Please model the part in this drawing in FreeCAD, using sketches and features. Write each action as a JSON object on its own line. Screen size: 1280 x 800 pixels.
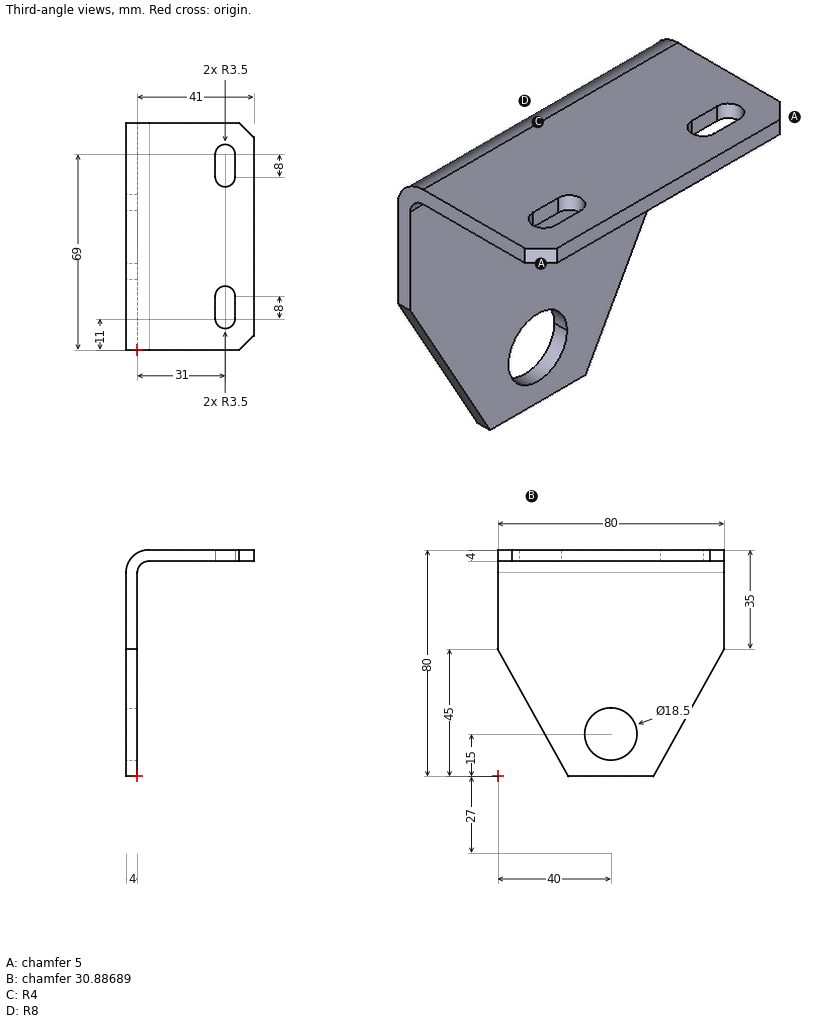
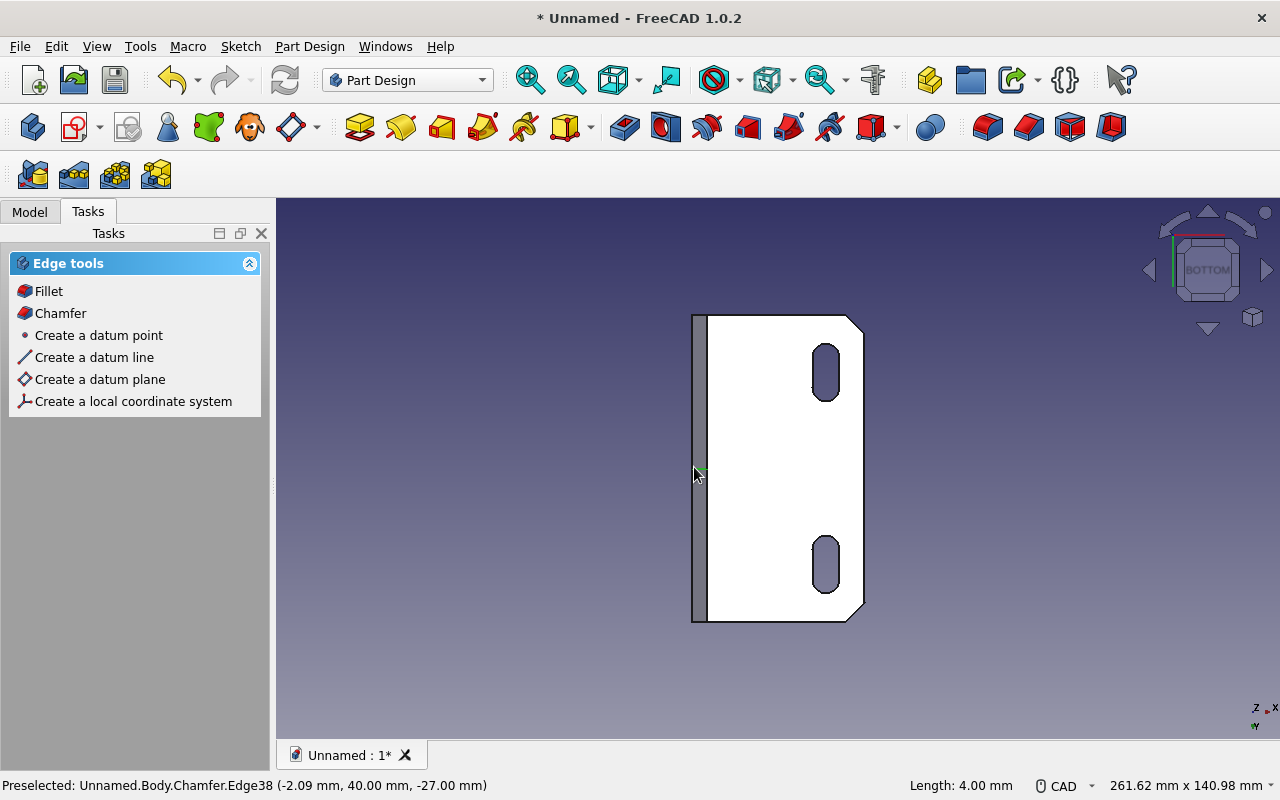
{"action": "left_click", "coordinate": [1029, 128]}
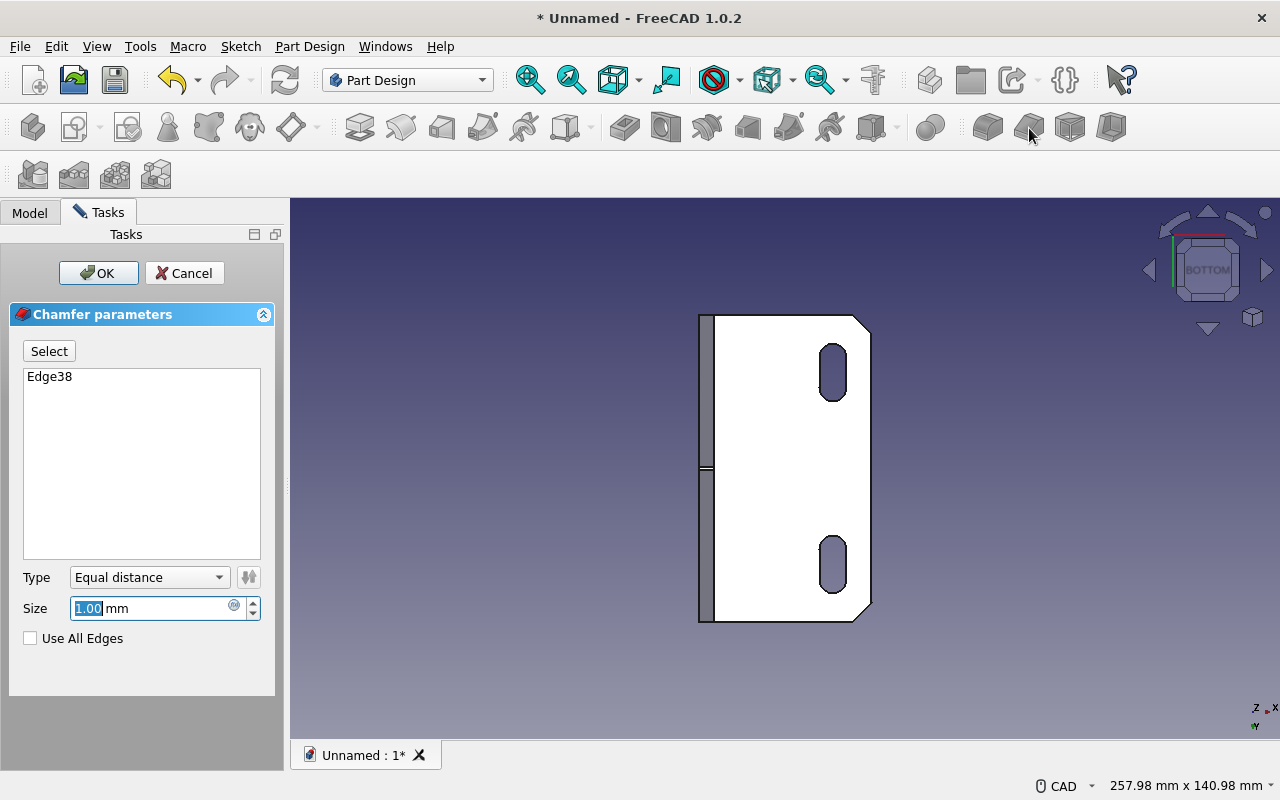
{"action": "type", "text": "30.88689"}
{"action": "key", "text": "Tab"}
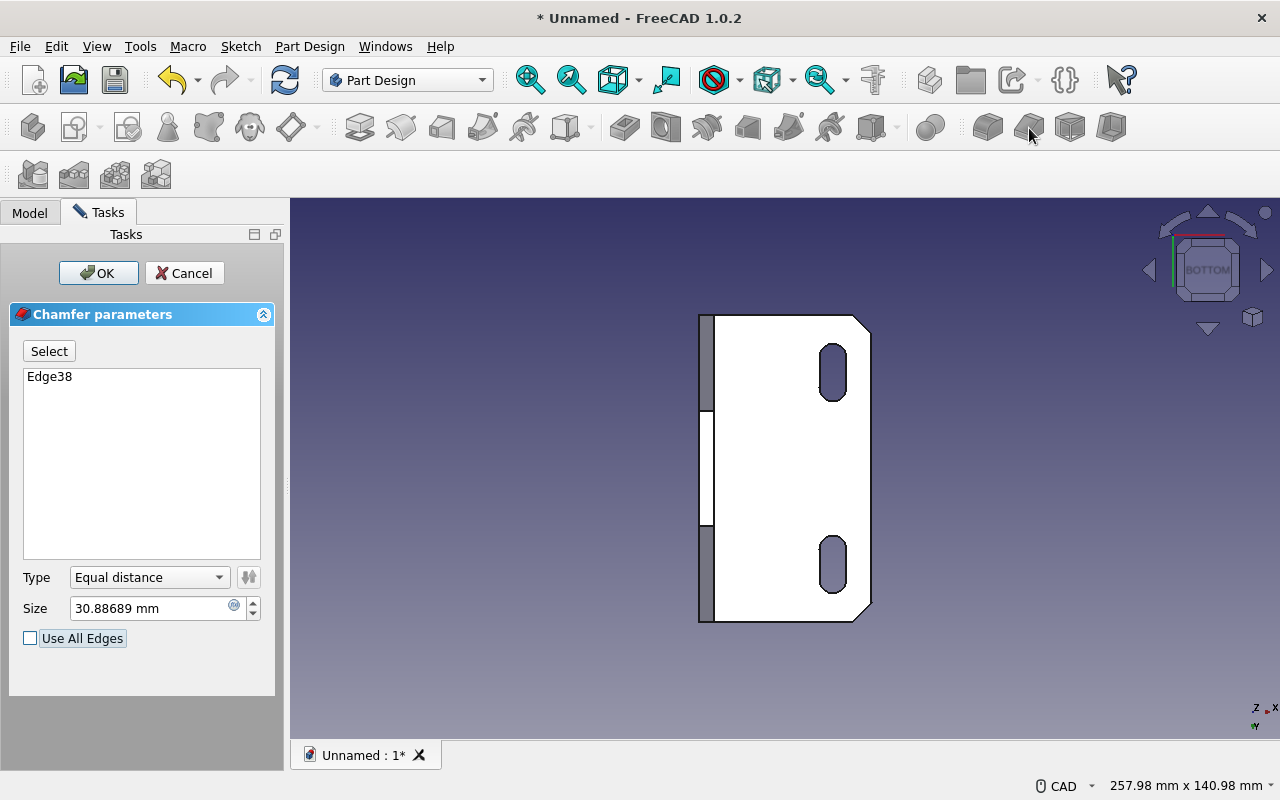
{"action": "left_click", "coordinate": [99, 273]}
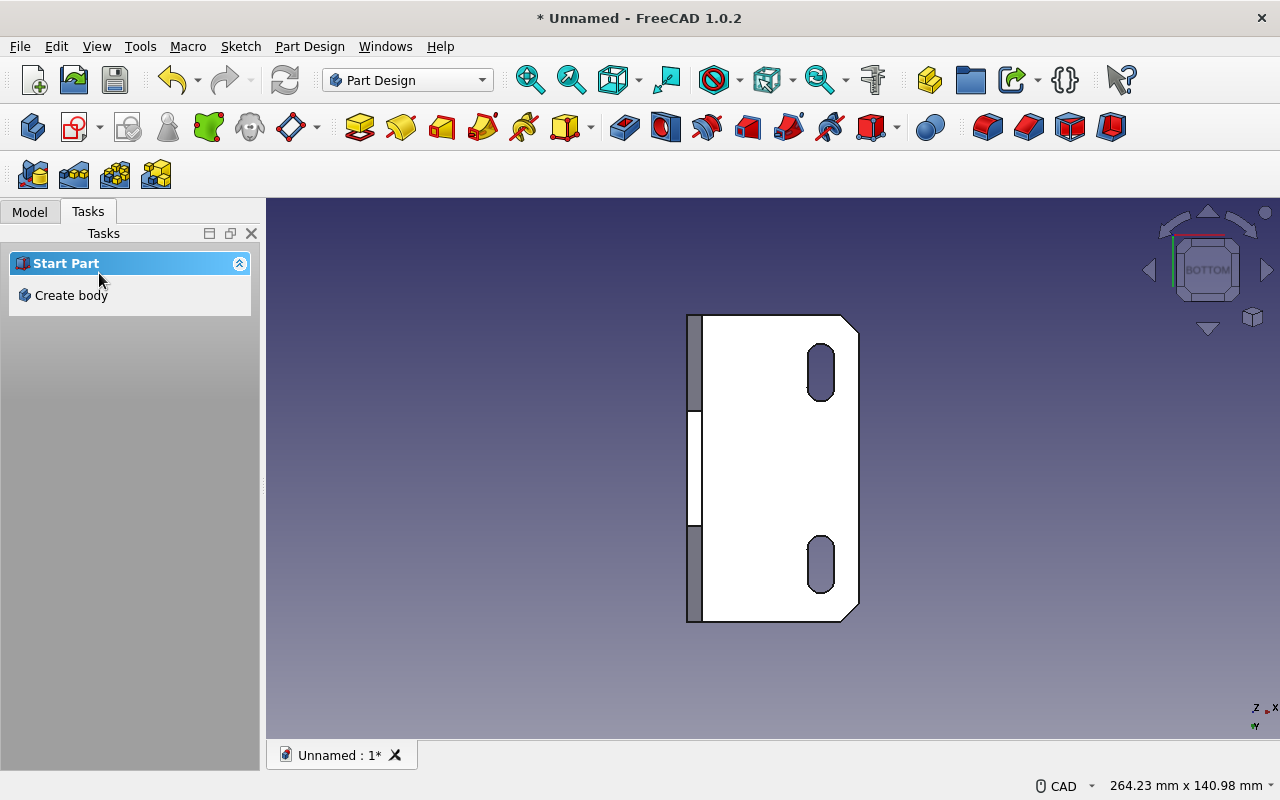
{"action": "key", "text": "0"}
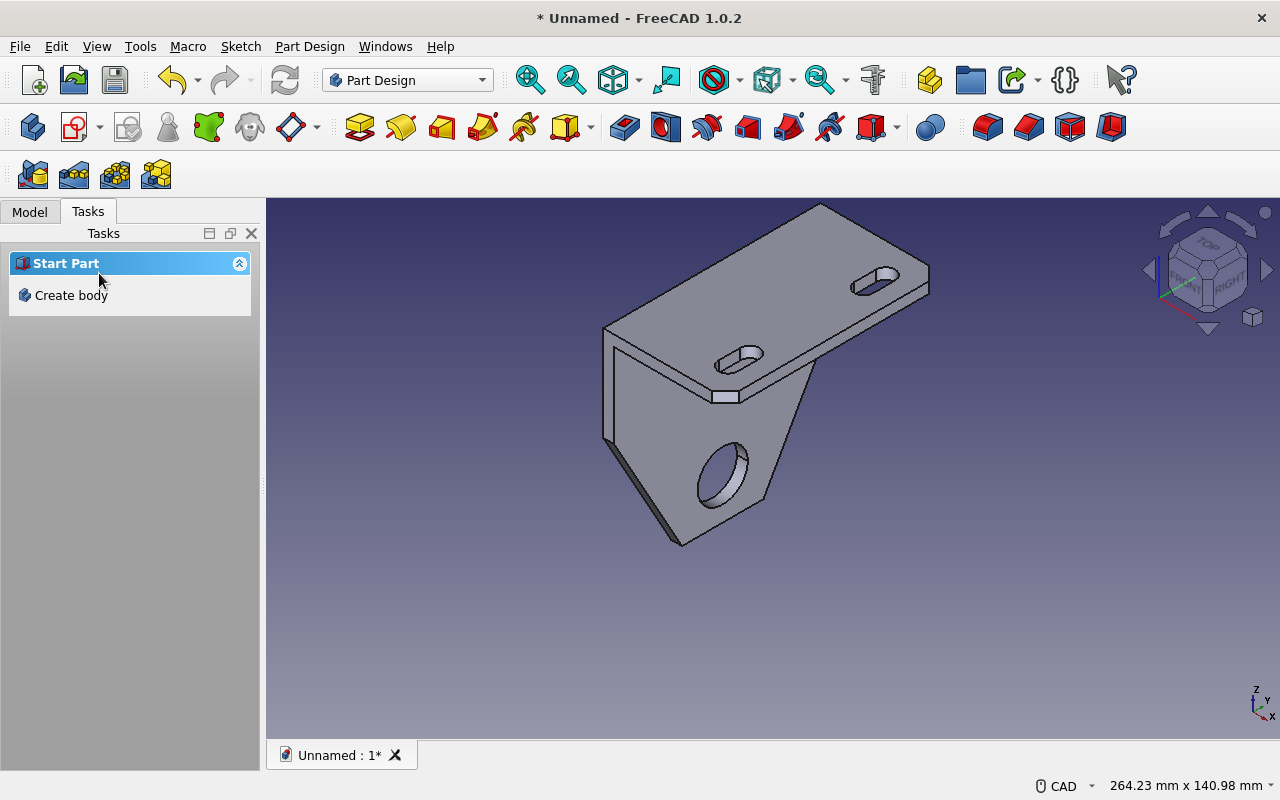
{"action": "key", "text": "2"}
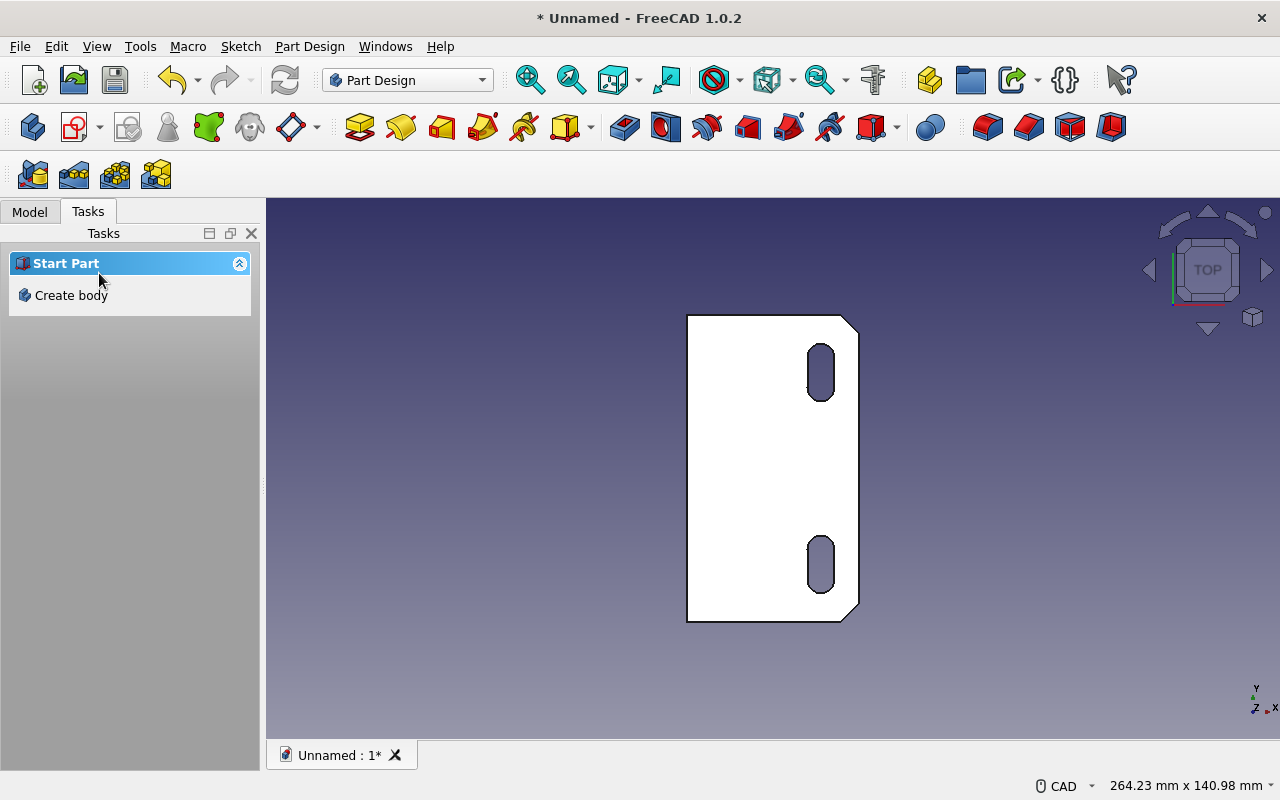
{"action": "key", "text": "1"}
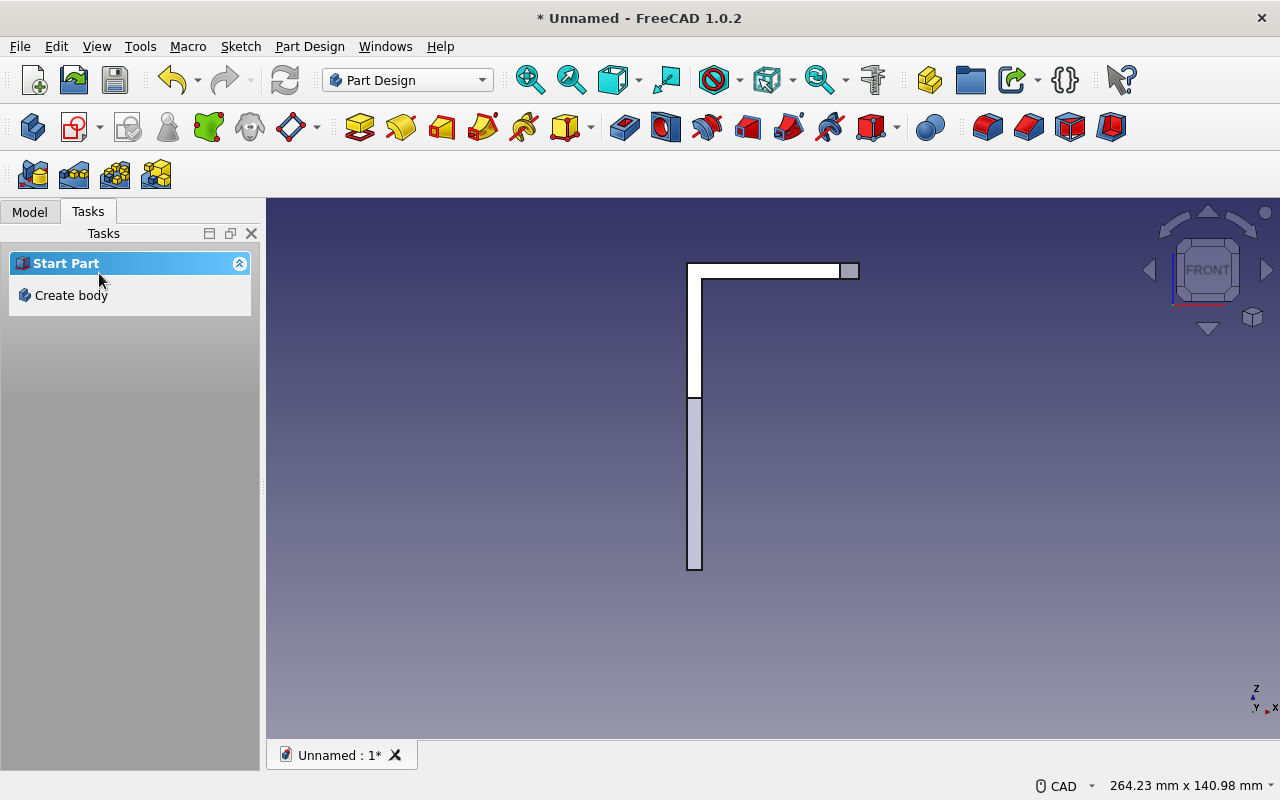
{"action": "key", "text": "3"}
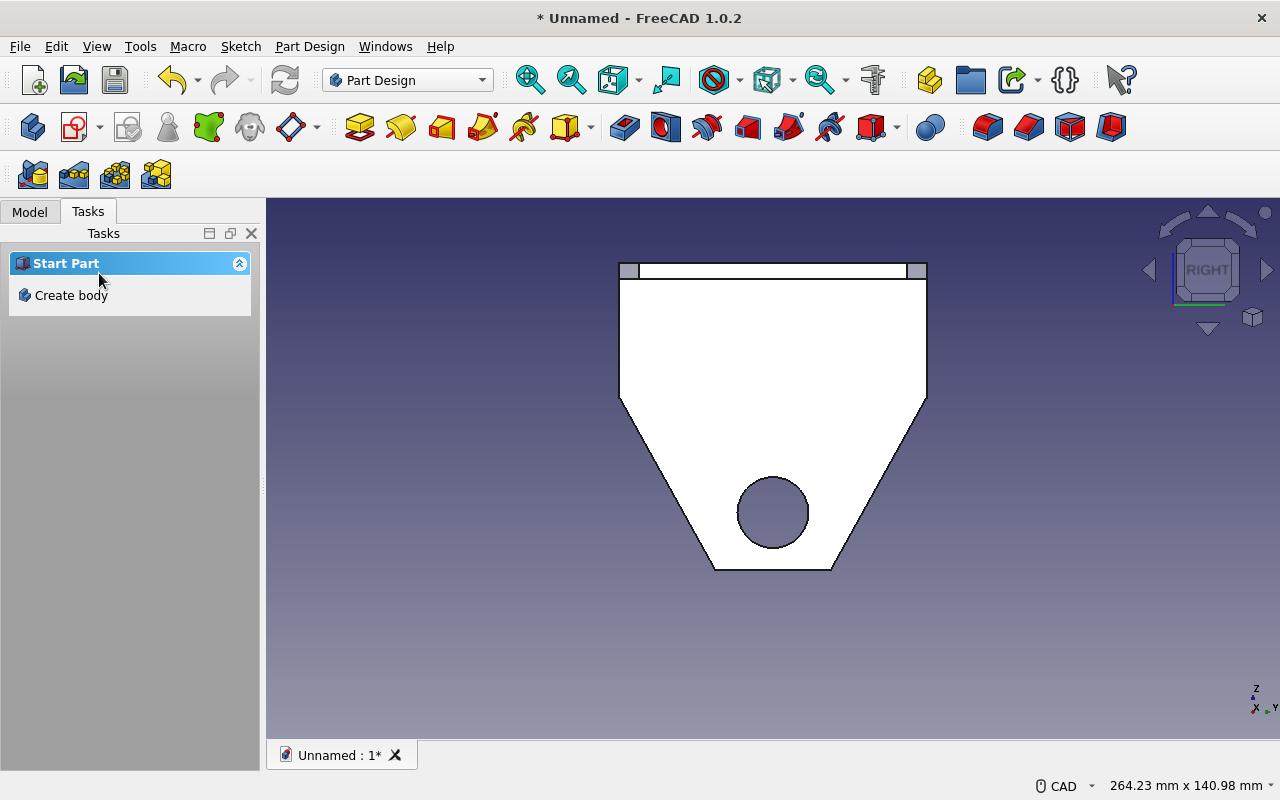
{"action": "key", "text": "5"}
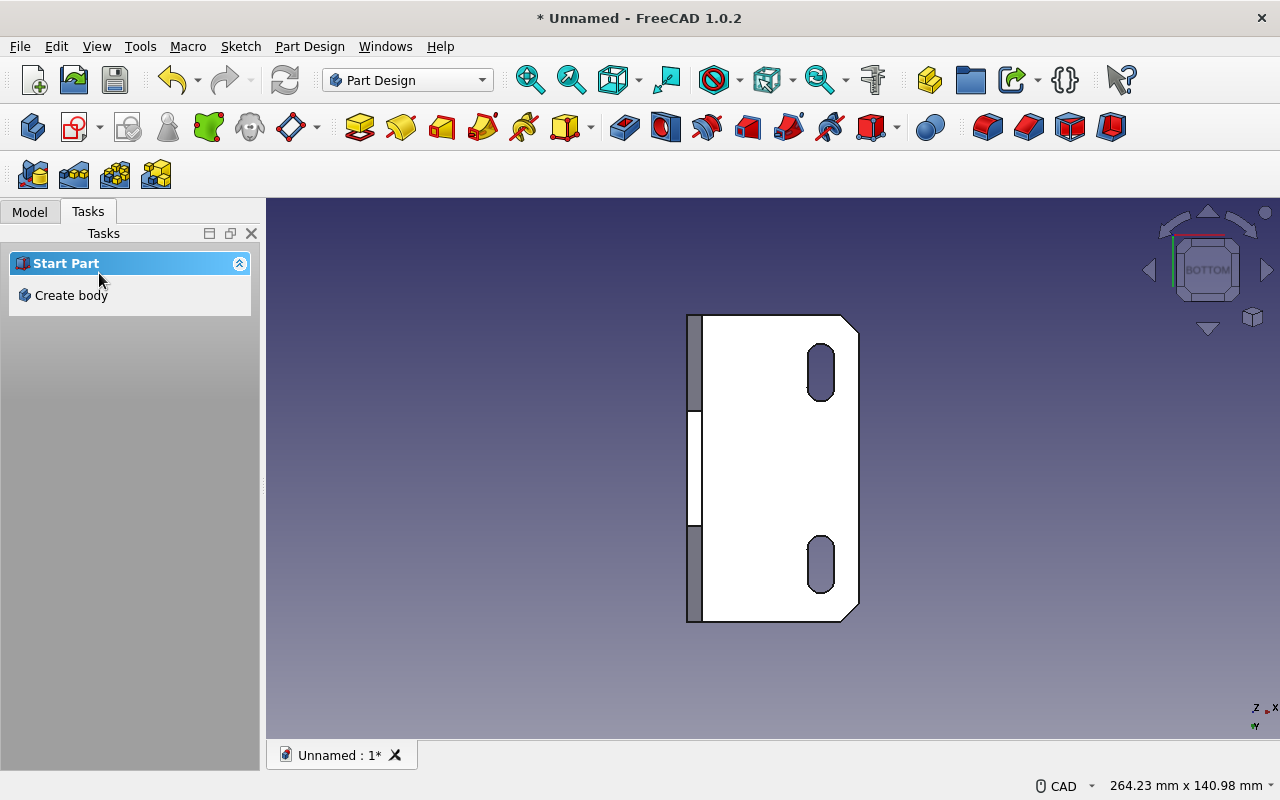
{"action": "key", "text": "4"}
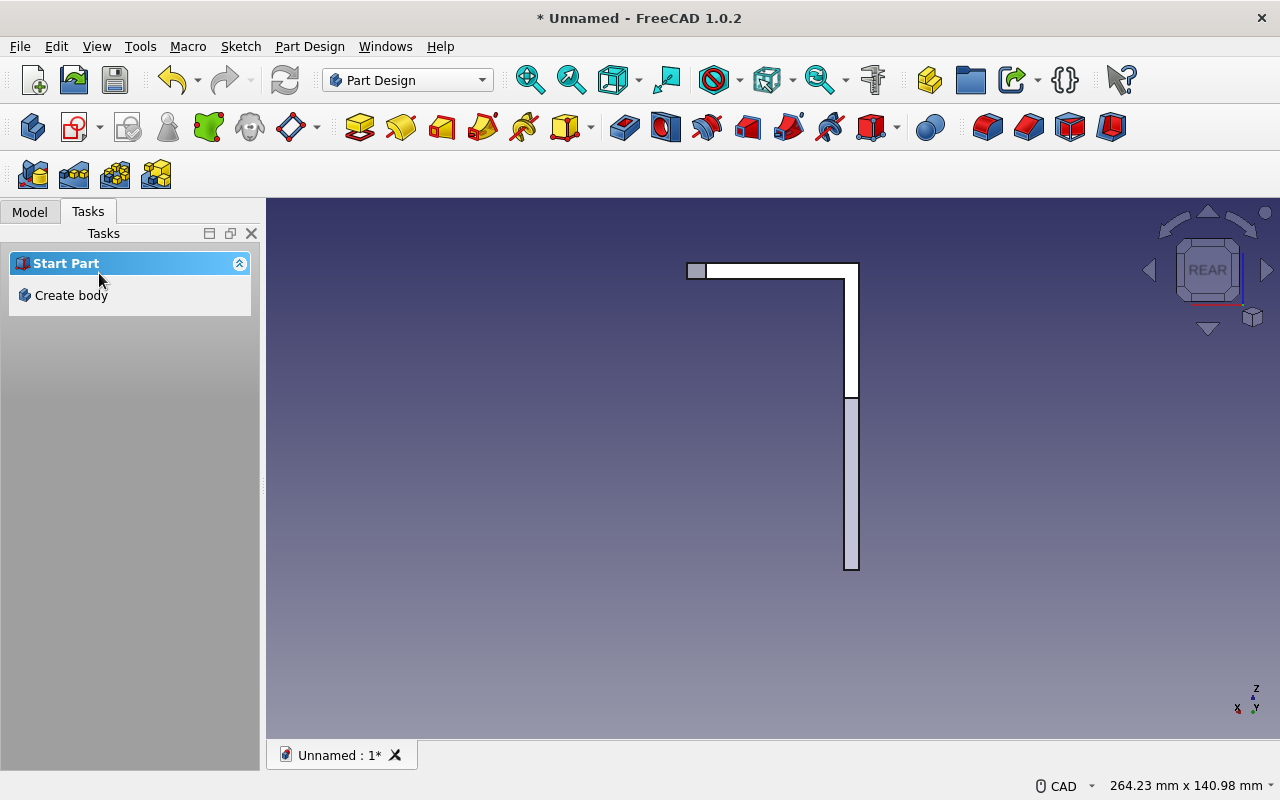
{"action": "key", "text": "6"}